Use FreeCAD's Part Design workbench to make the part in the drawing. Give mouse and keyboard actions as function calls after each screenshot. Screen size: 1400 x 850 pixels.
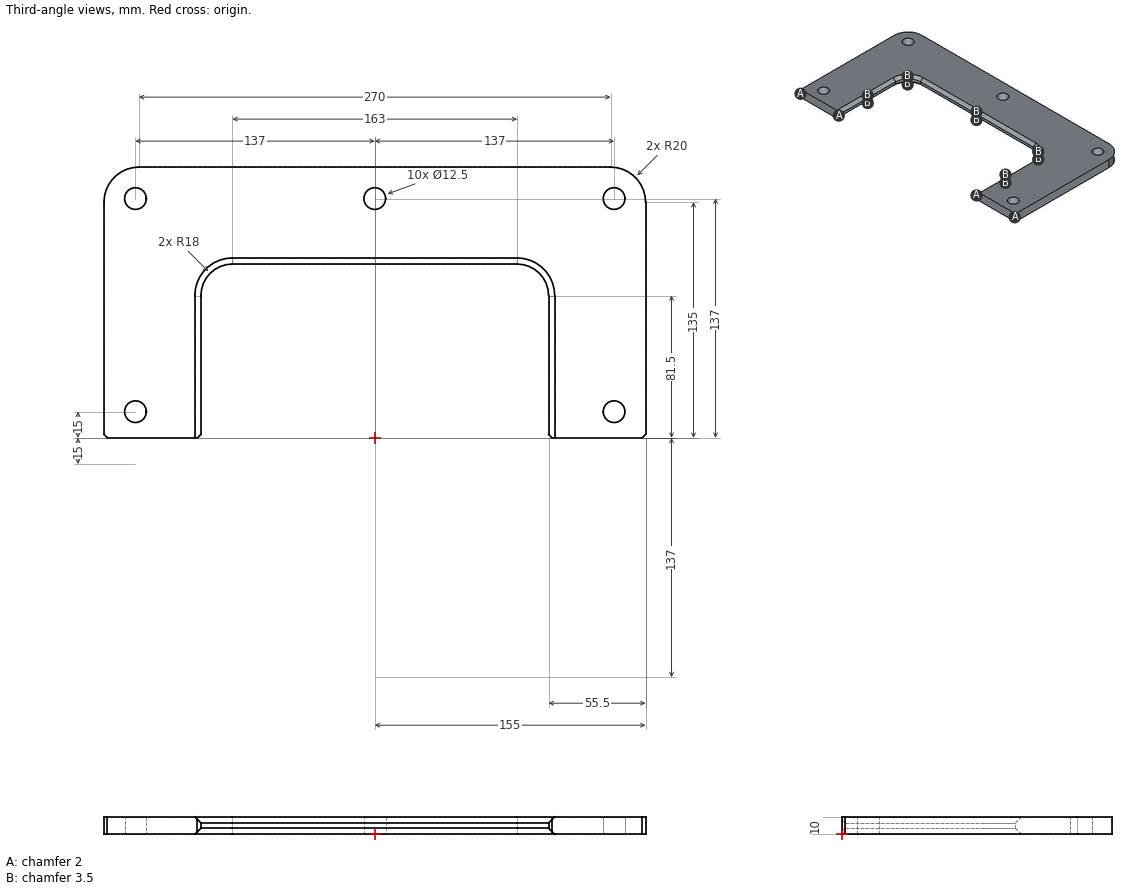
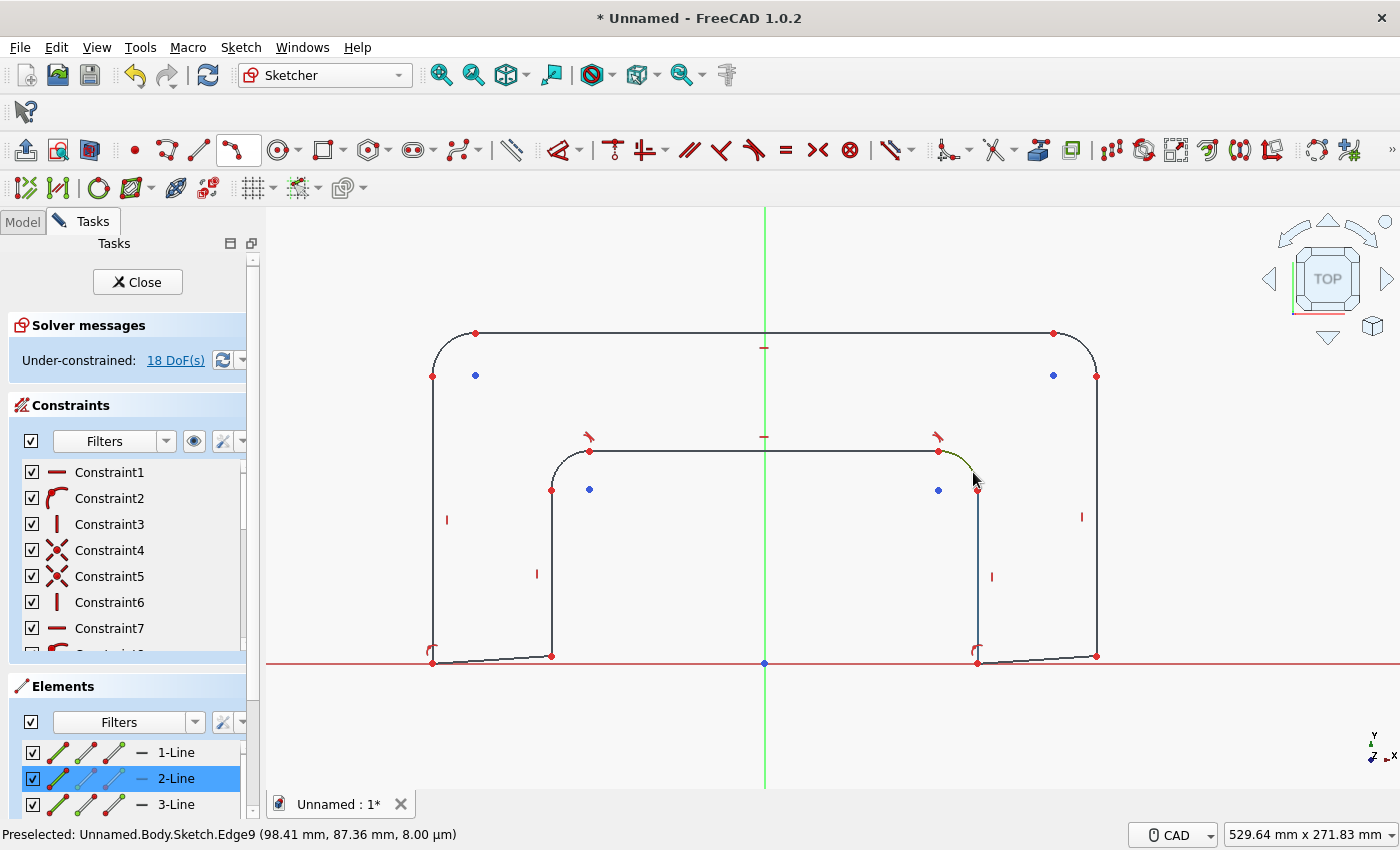
key(t)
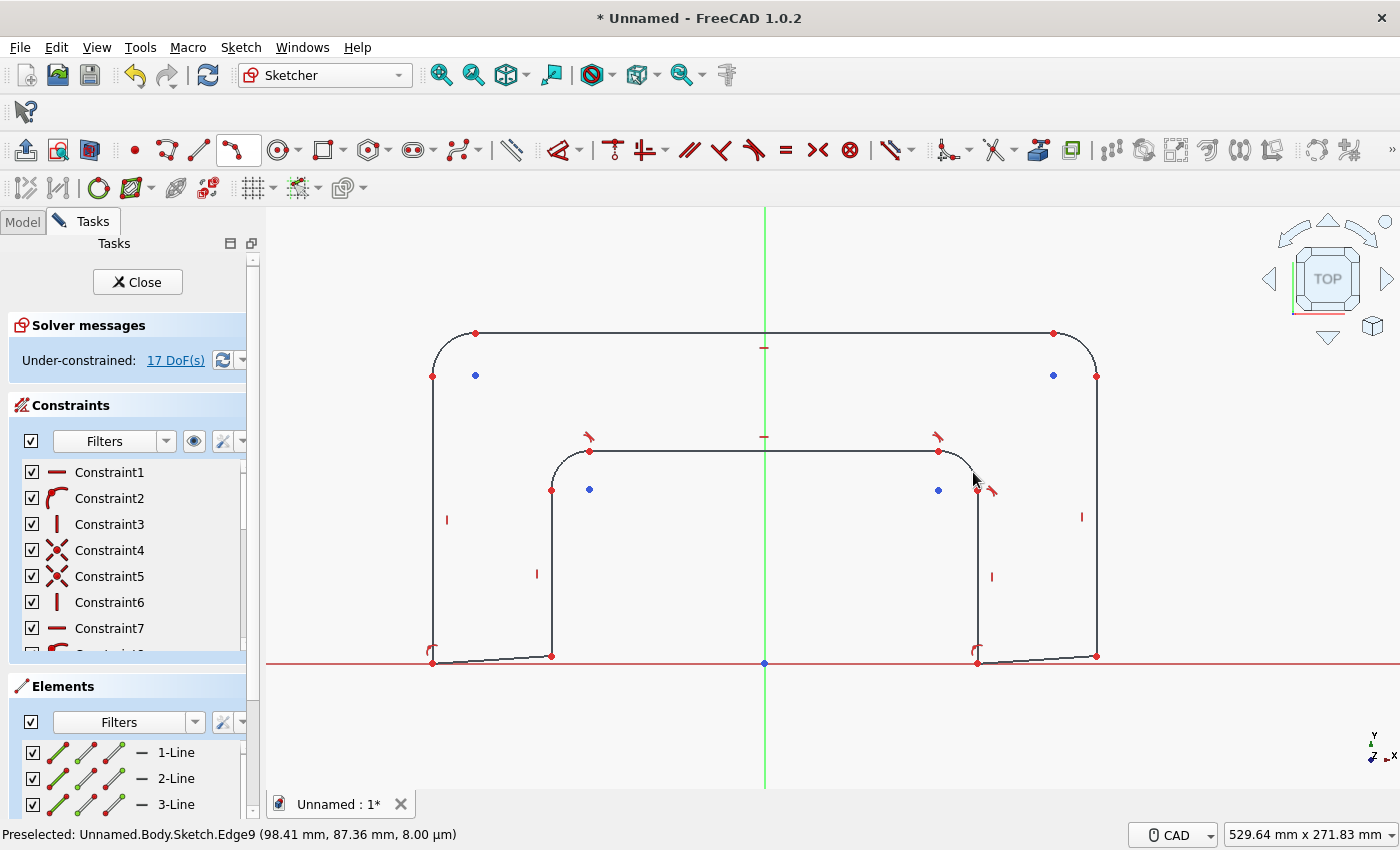
click(1097, 572)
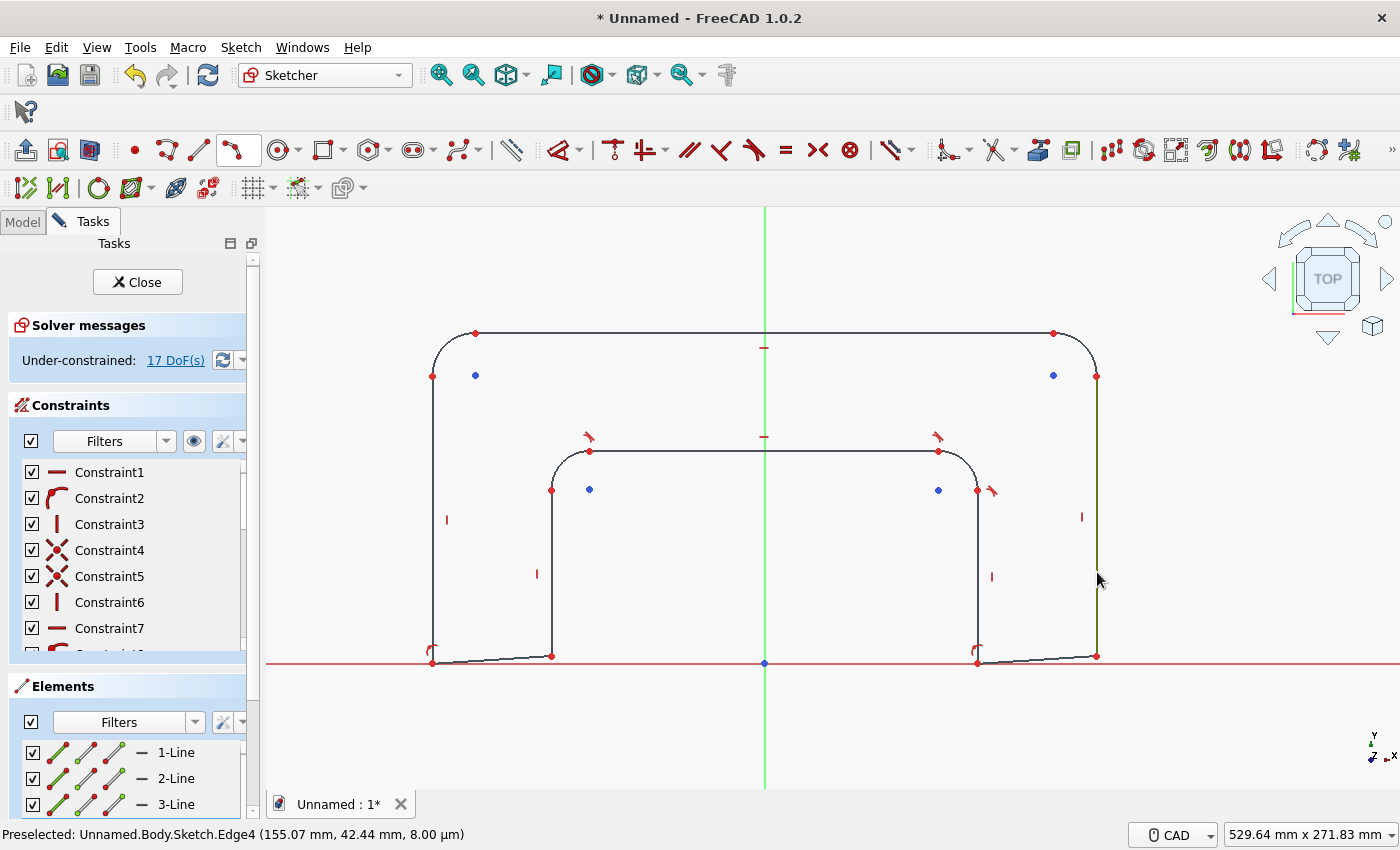
click(1092, 356)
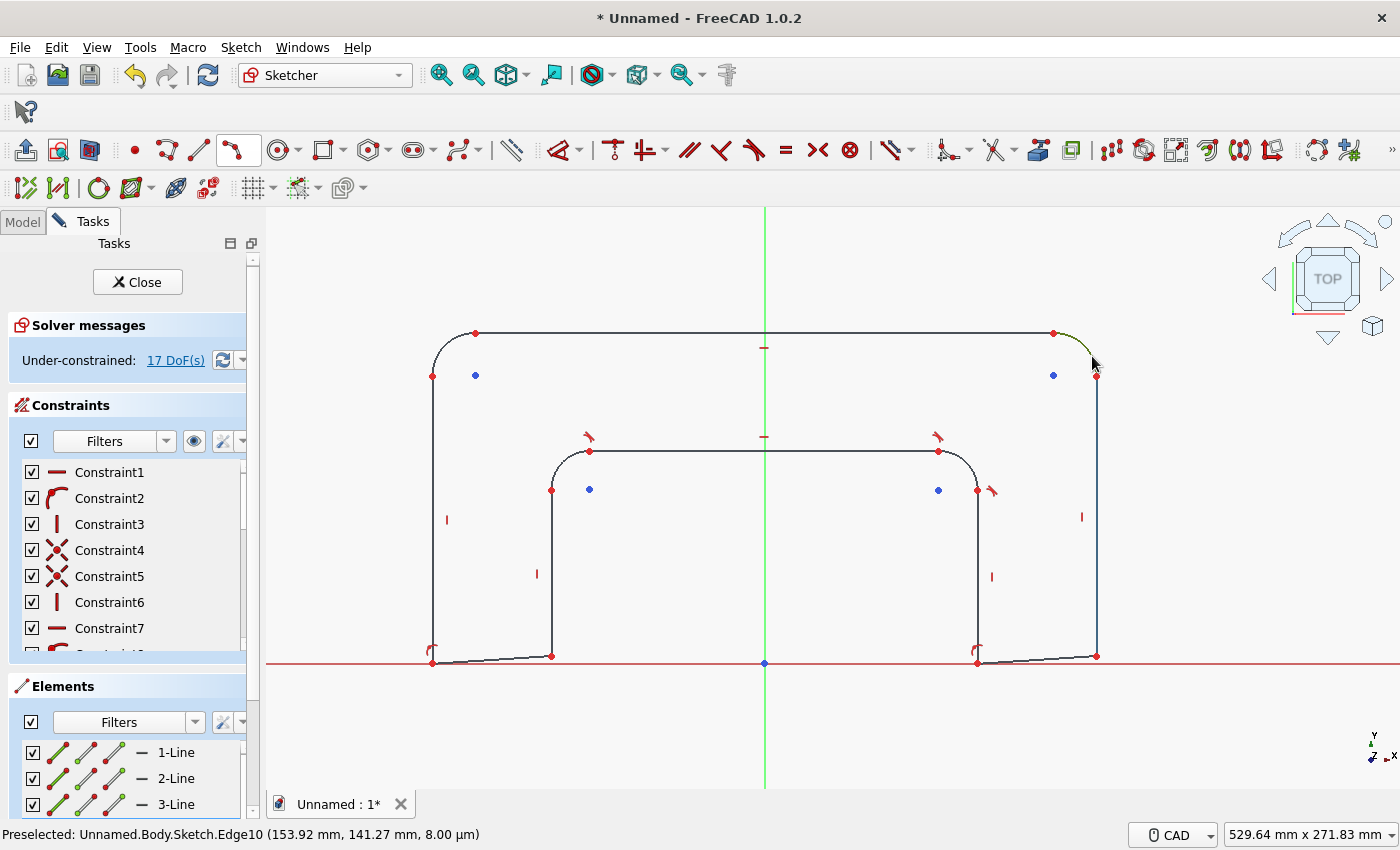
key(t)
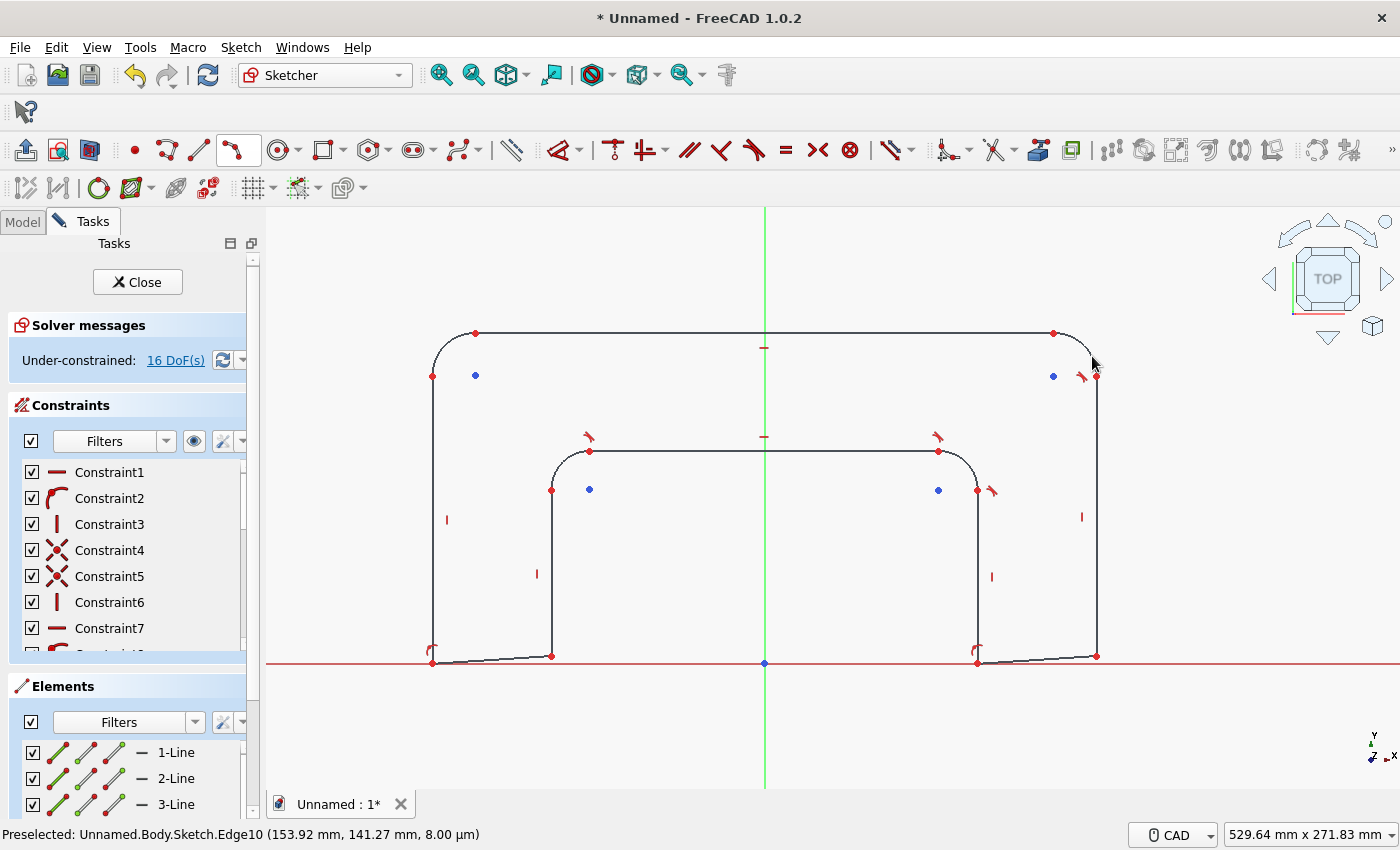
click(880, 333)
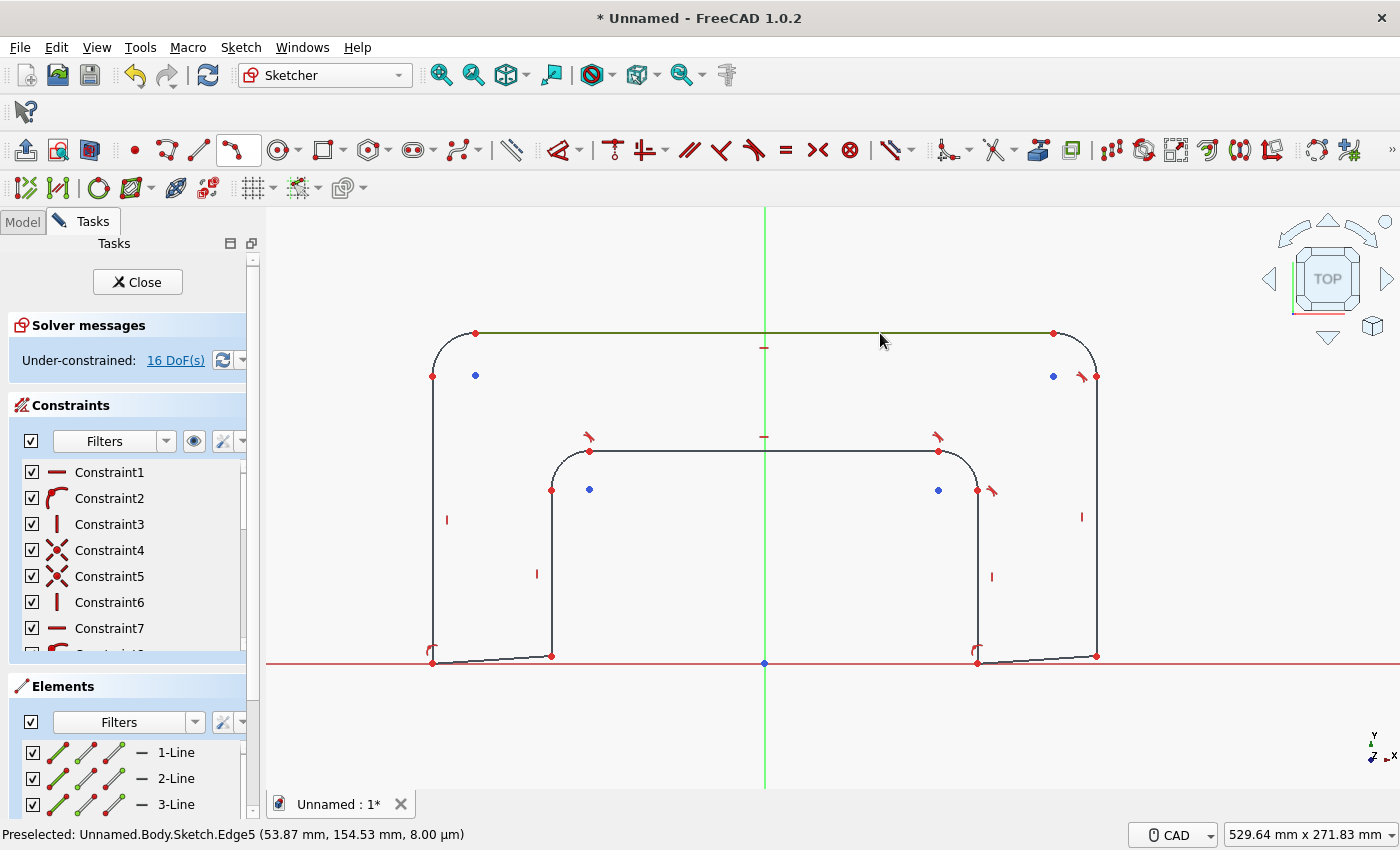
click(1092, 356)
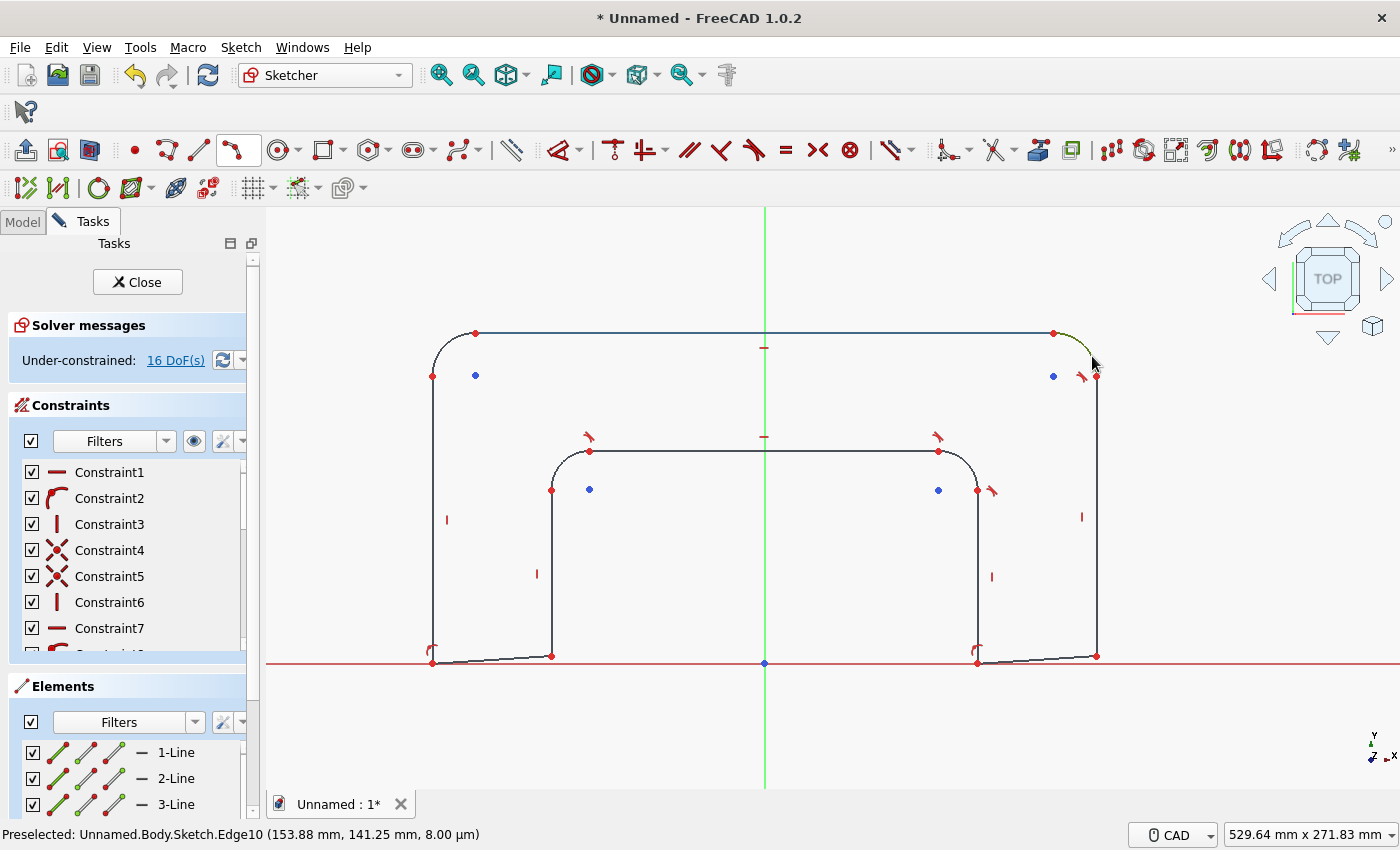
key(t)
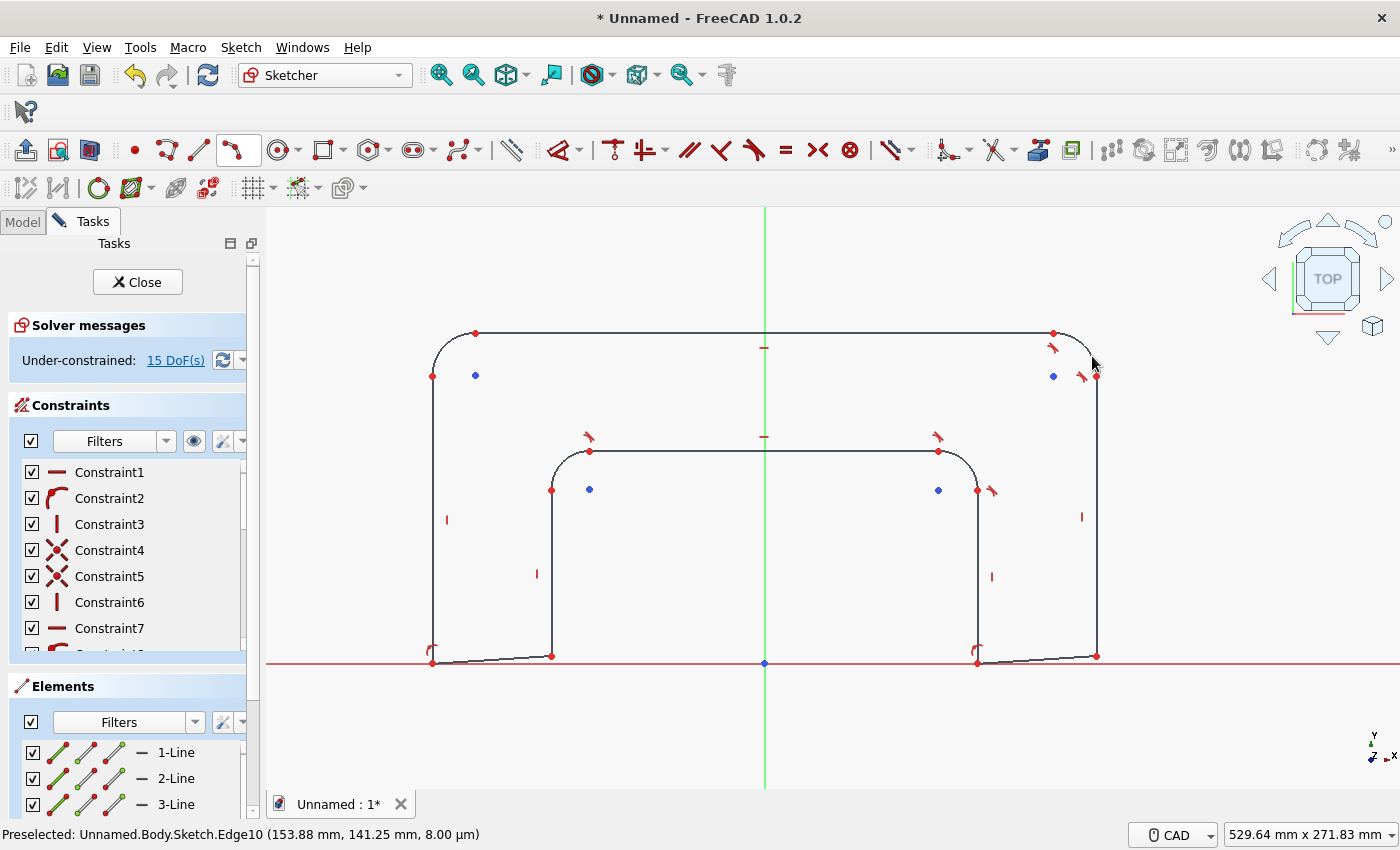
click(880, 333)